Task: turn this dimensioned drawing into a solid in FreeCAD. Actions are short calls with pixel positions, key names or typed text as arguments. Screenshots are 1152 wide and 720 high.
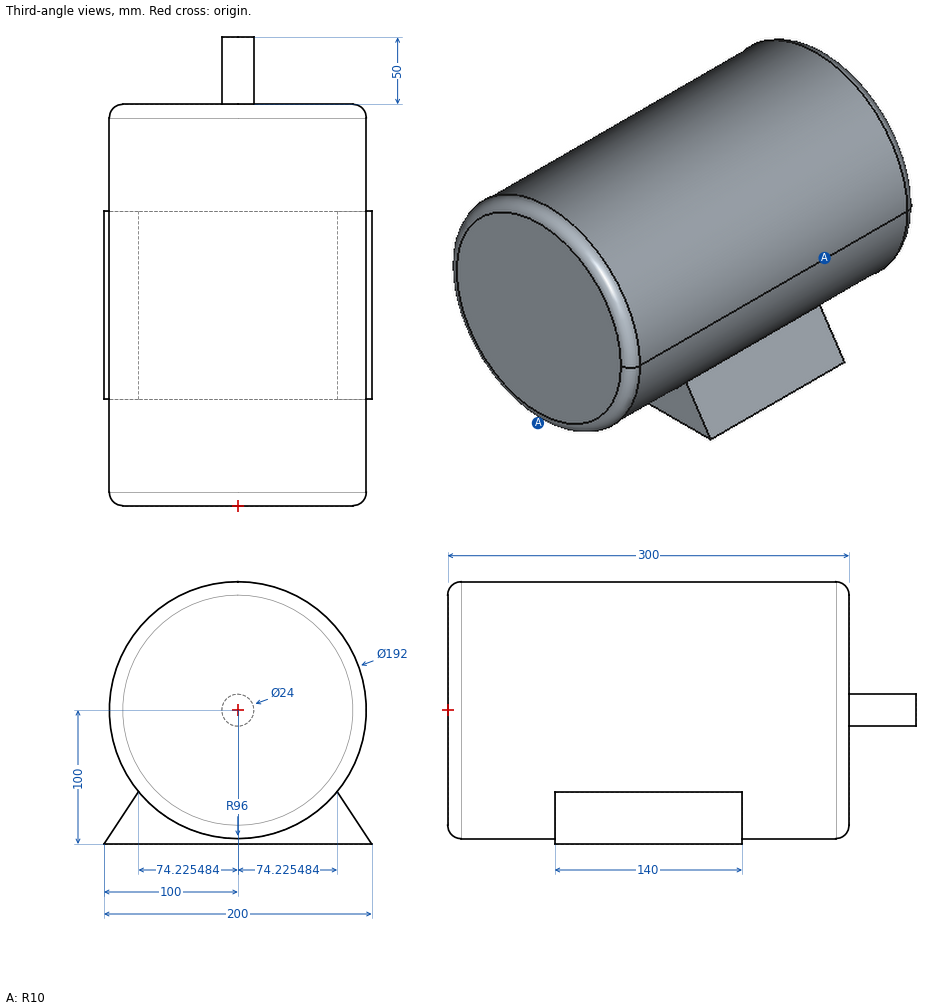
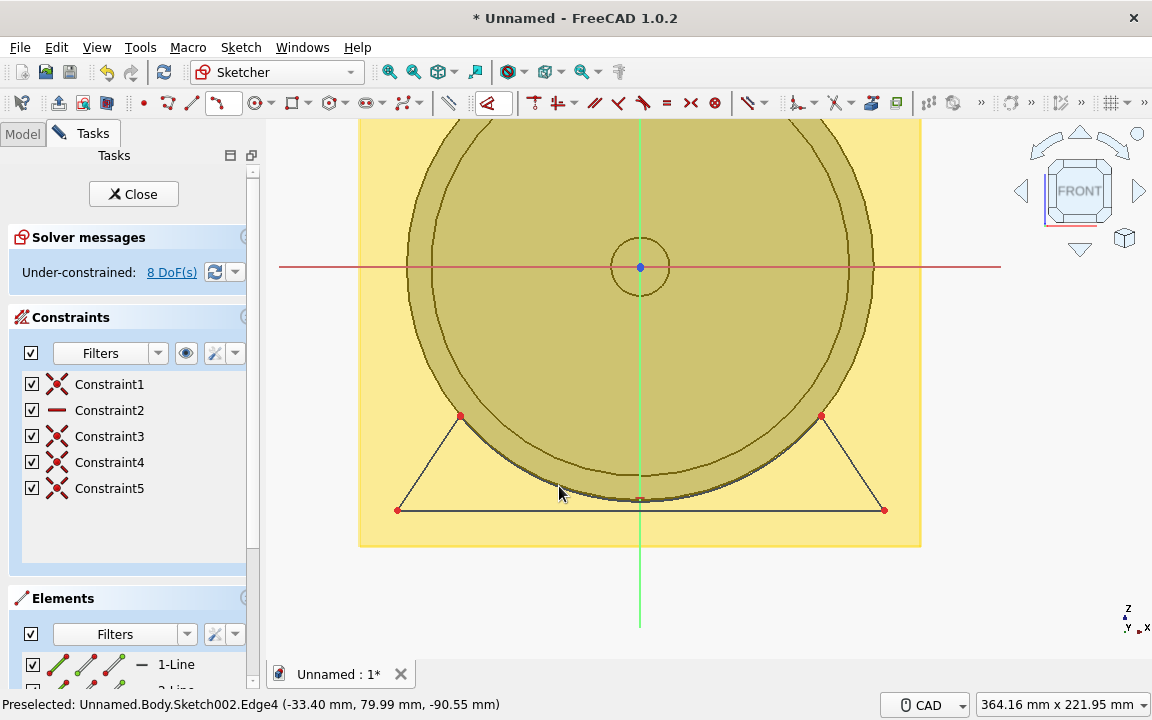
drag(630, 257, 651, 279)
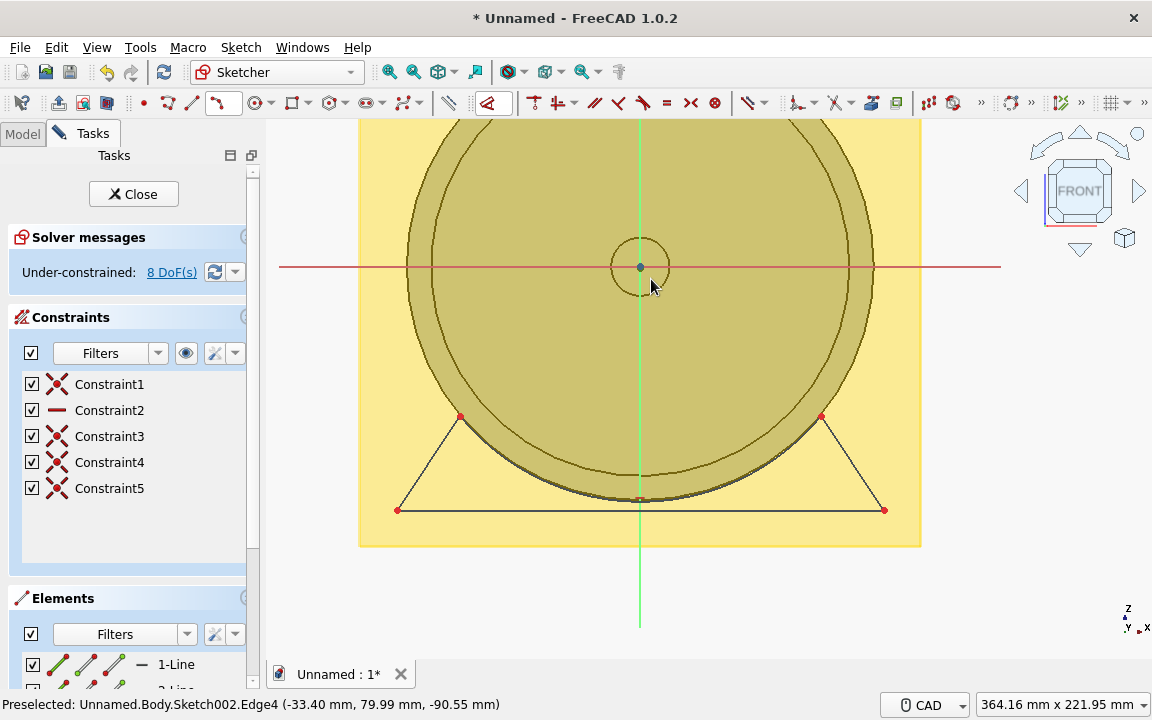
click(534, 104)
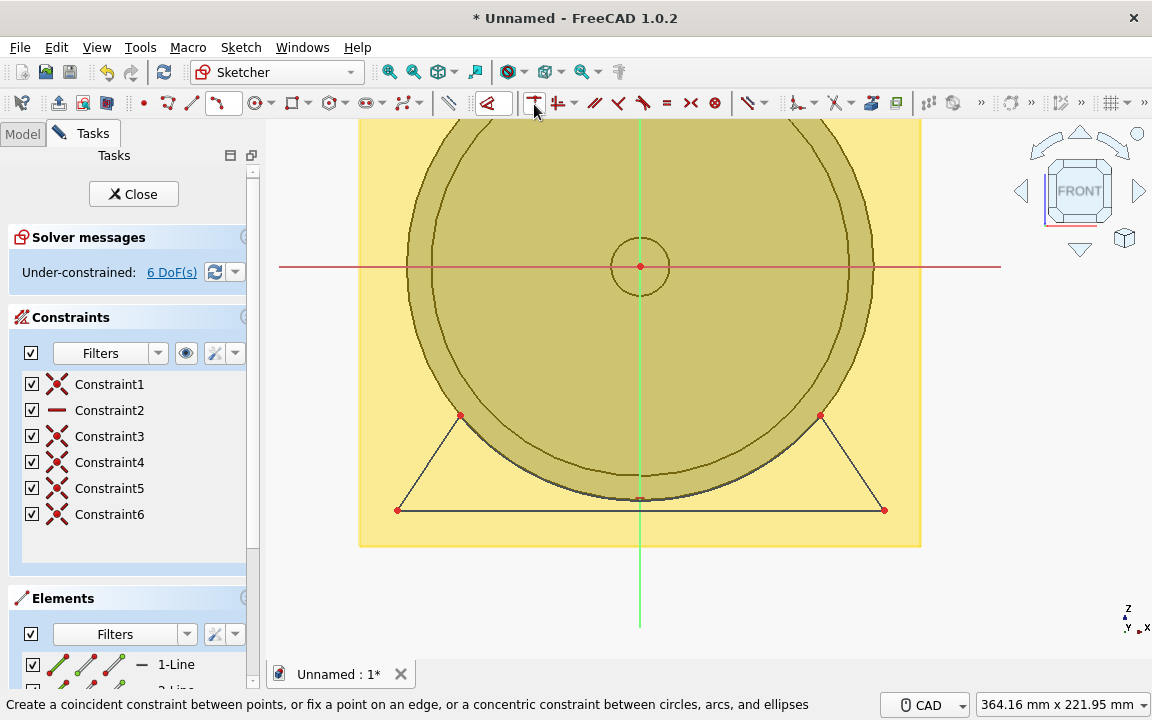
click(488, 104)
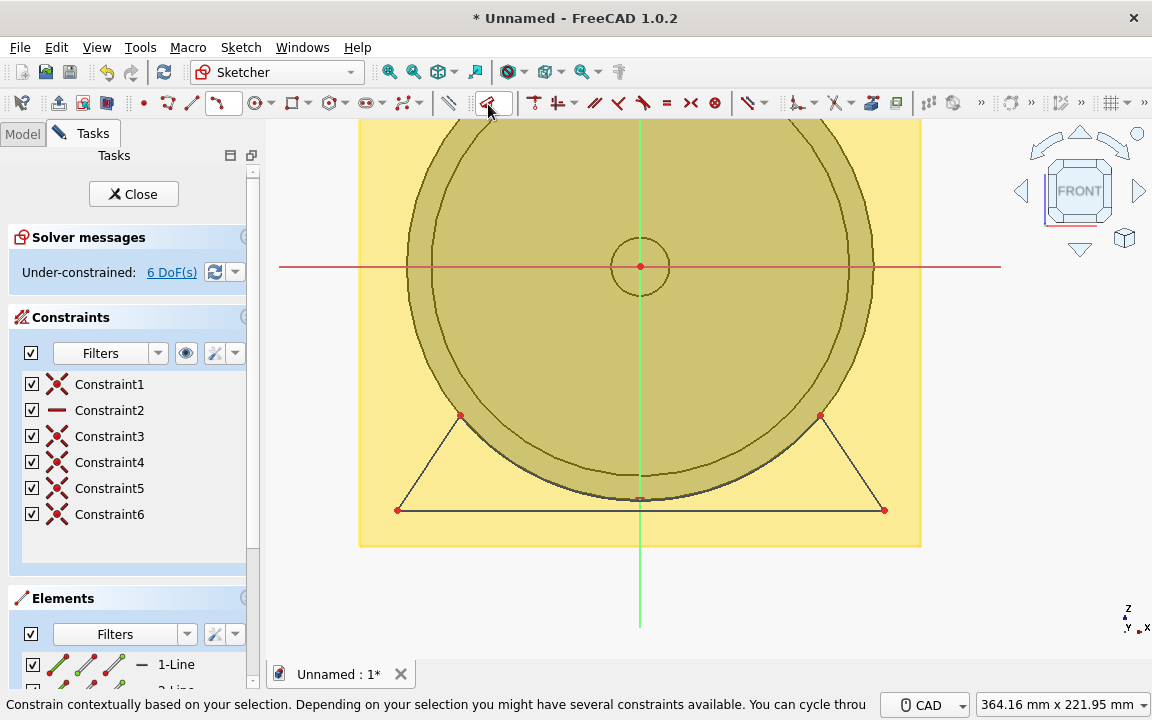
click(560, 486)
click(680, 529)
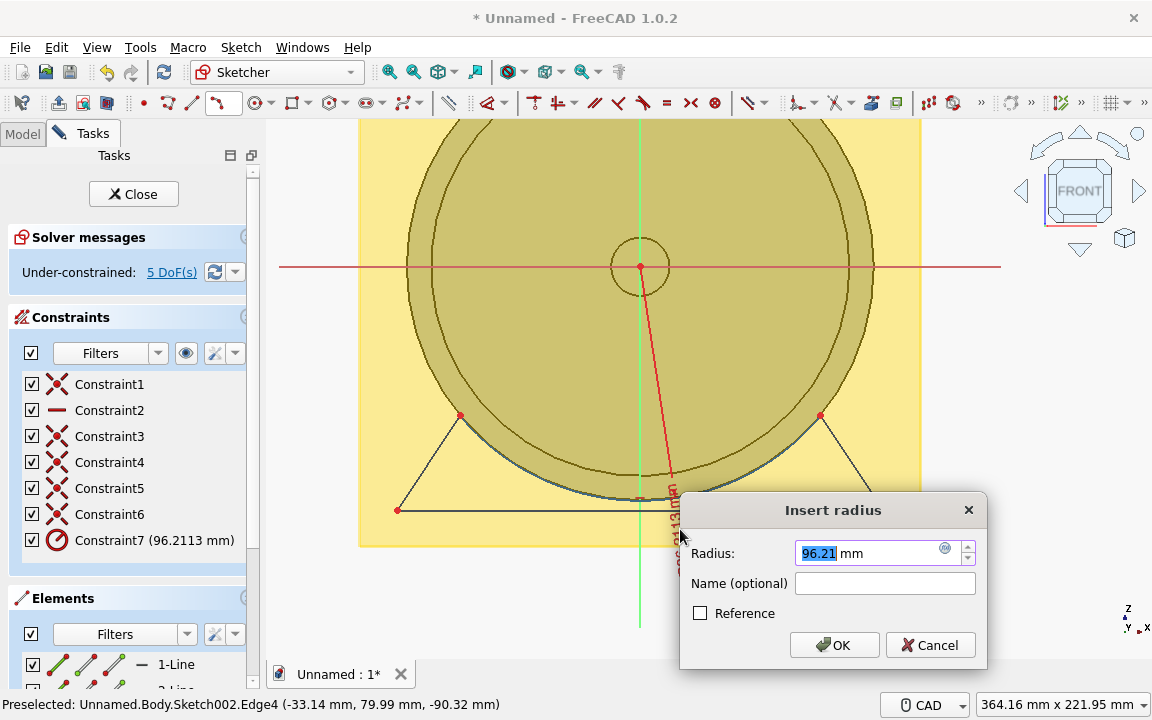
text(96)
key(Return)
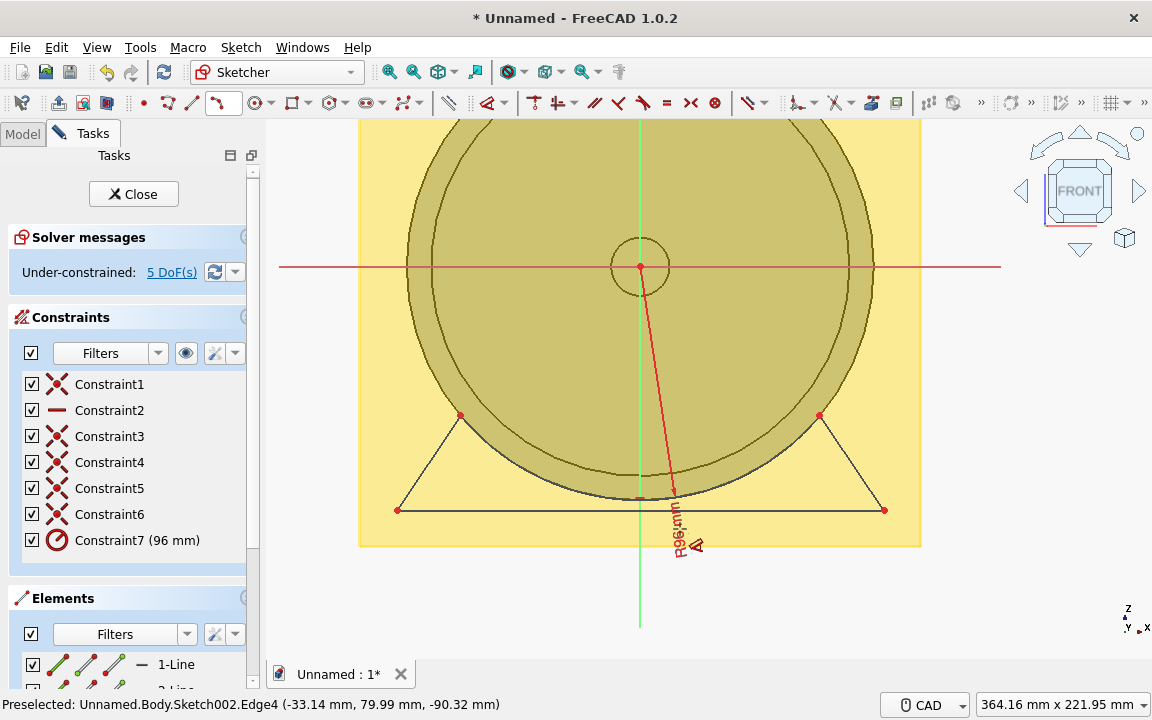
click(543, 511)
click(528, 545)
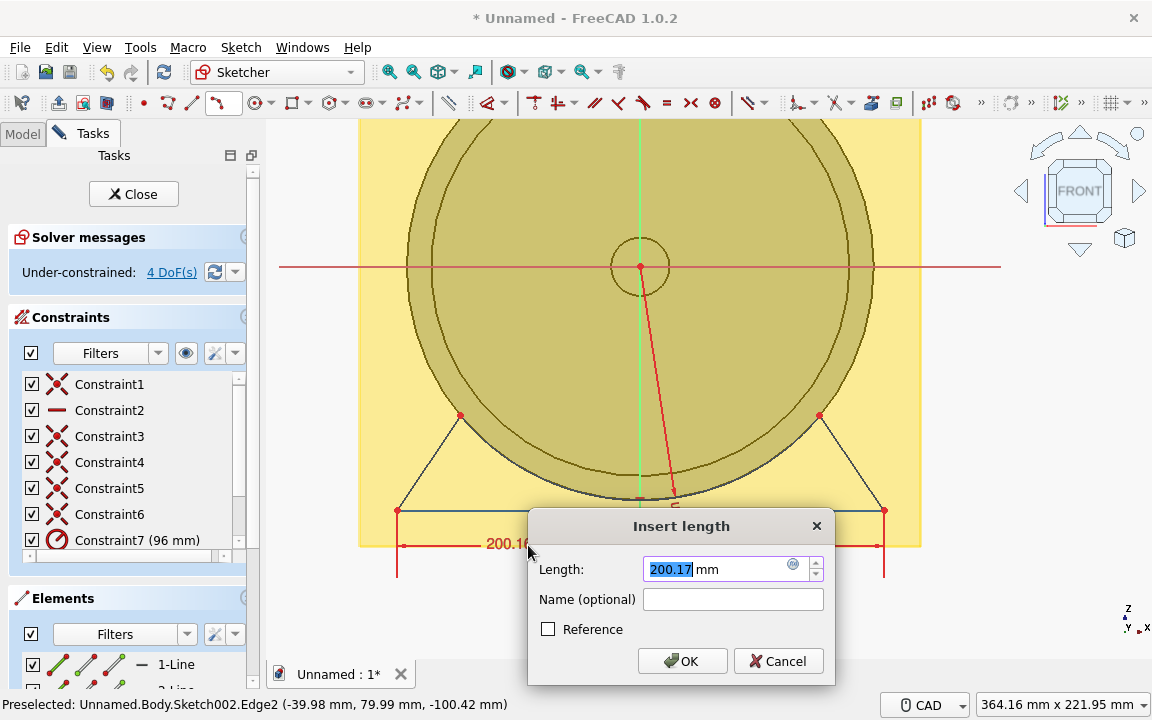
text(200)
key(Return)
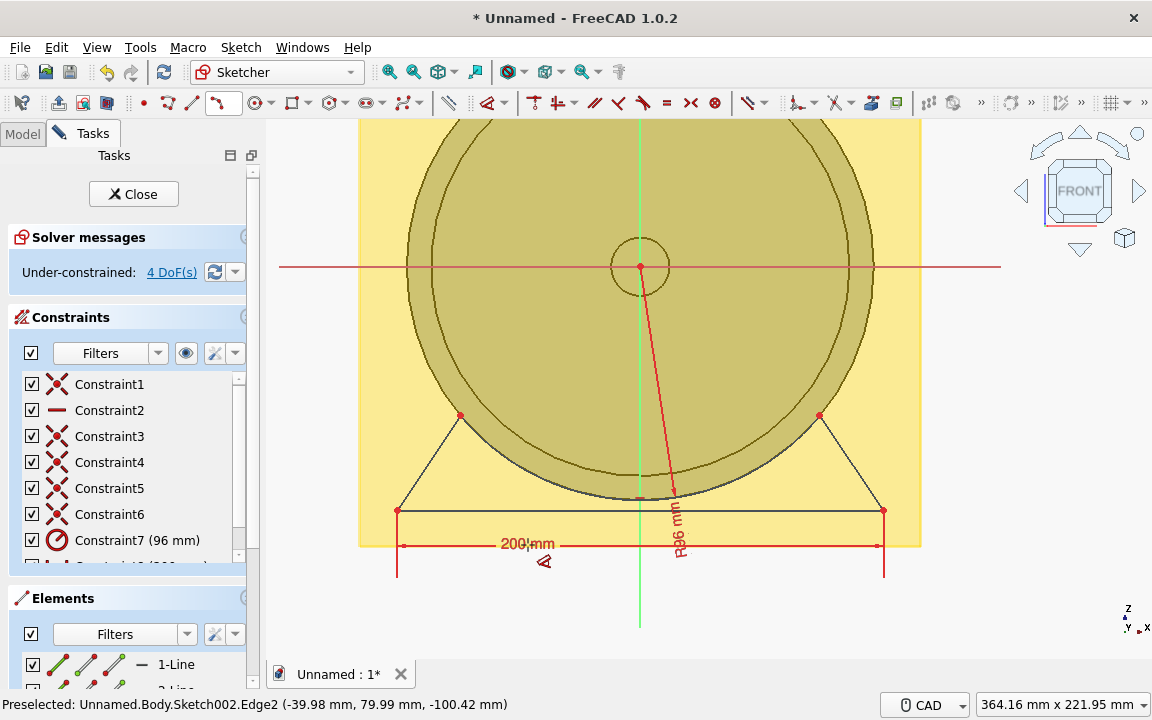
click(397, 511)
click(434, 545)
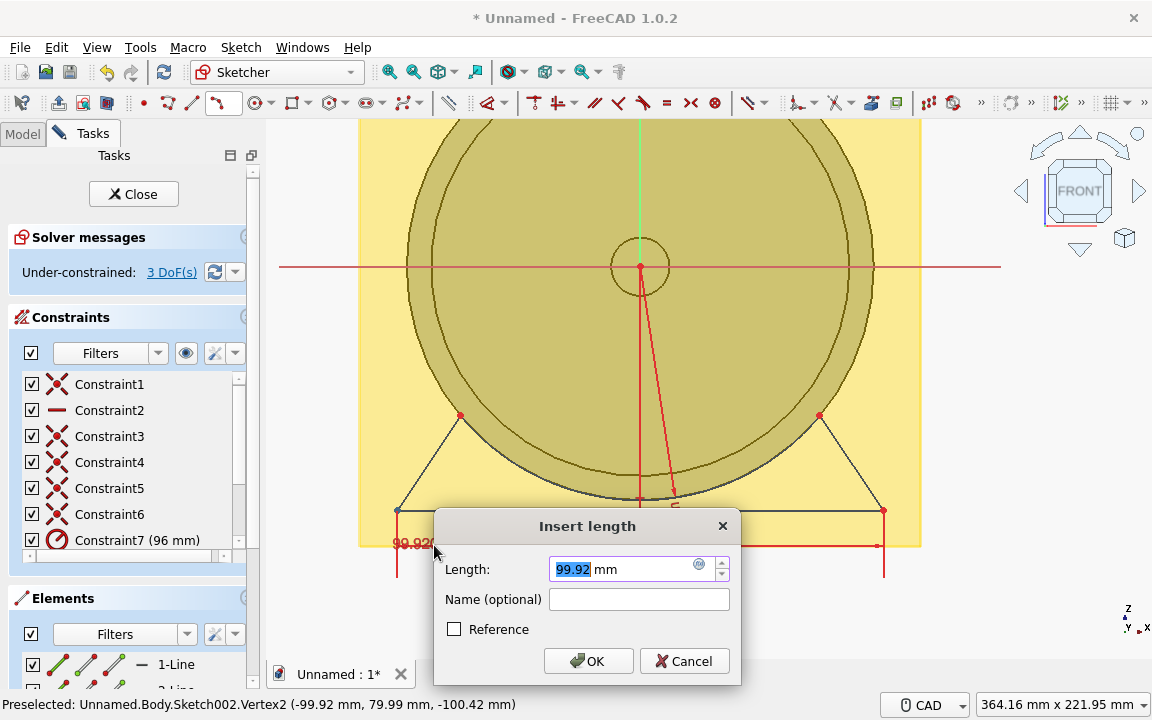
text(100)
key(Return)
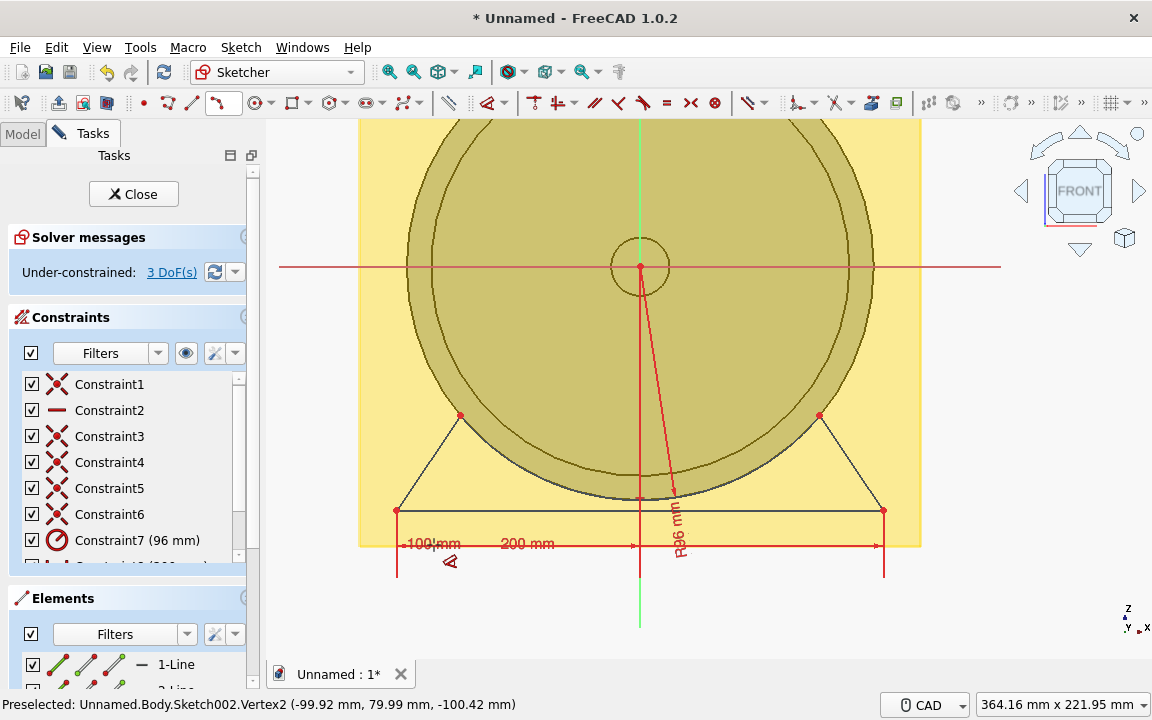
click(397, 511)
click(363, 389)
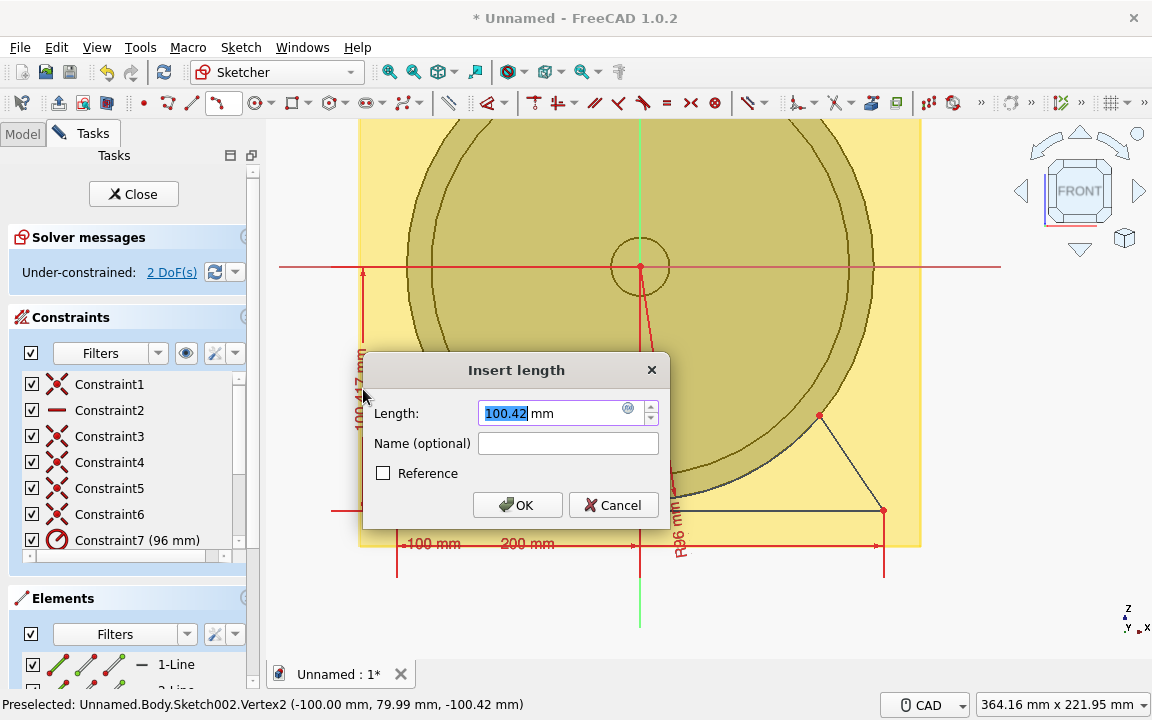
text(100)
key(Return)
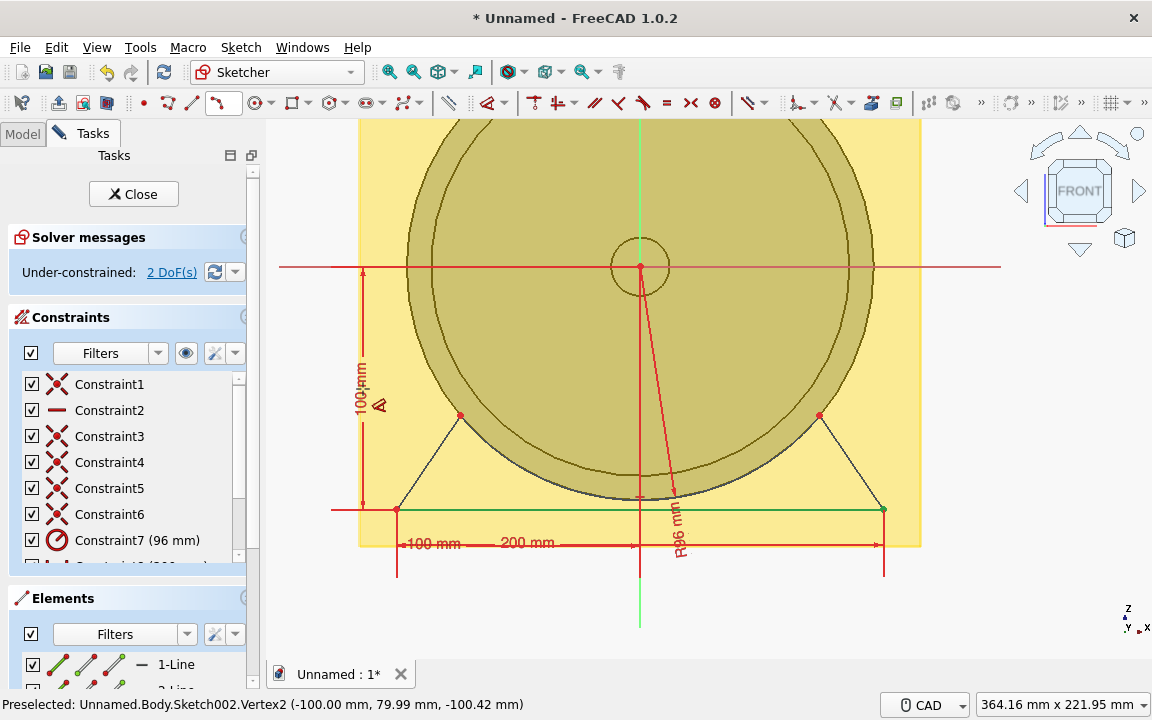
click(461, 416)
click(550, 233)